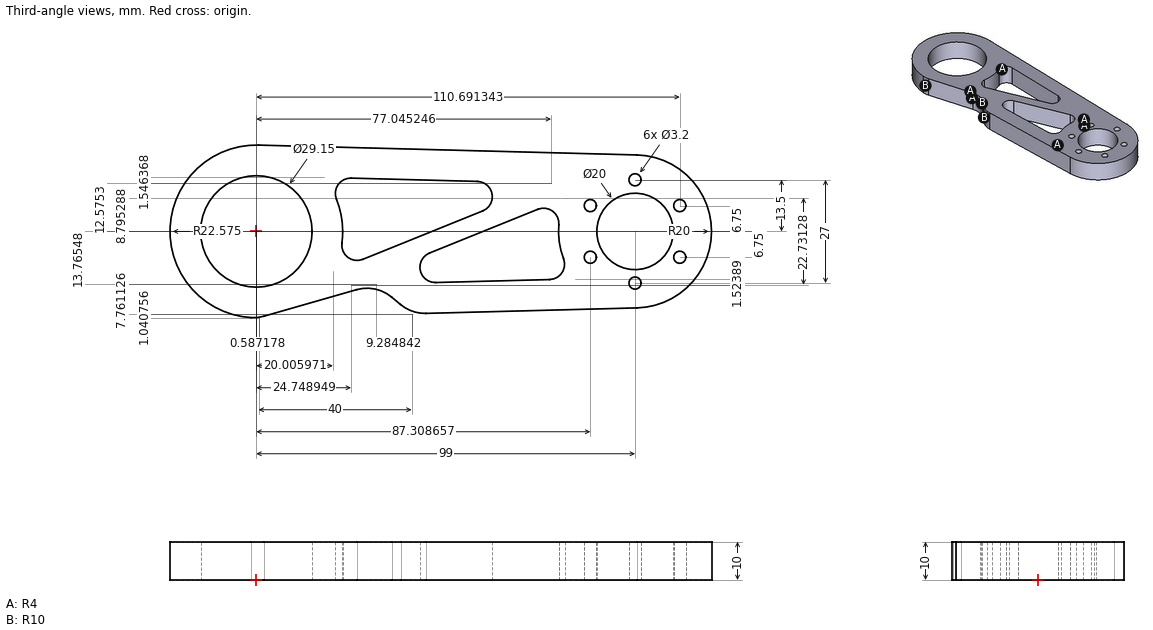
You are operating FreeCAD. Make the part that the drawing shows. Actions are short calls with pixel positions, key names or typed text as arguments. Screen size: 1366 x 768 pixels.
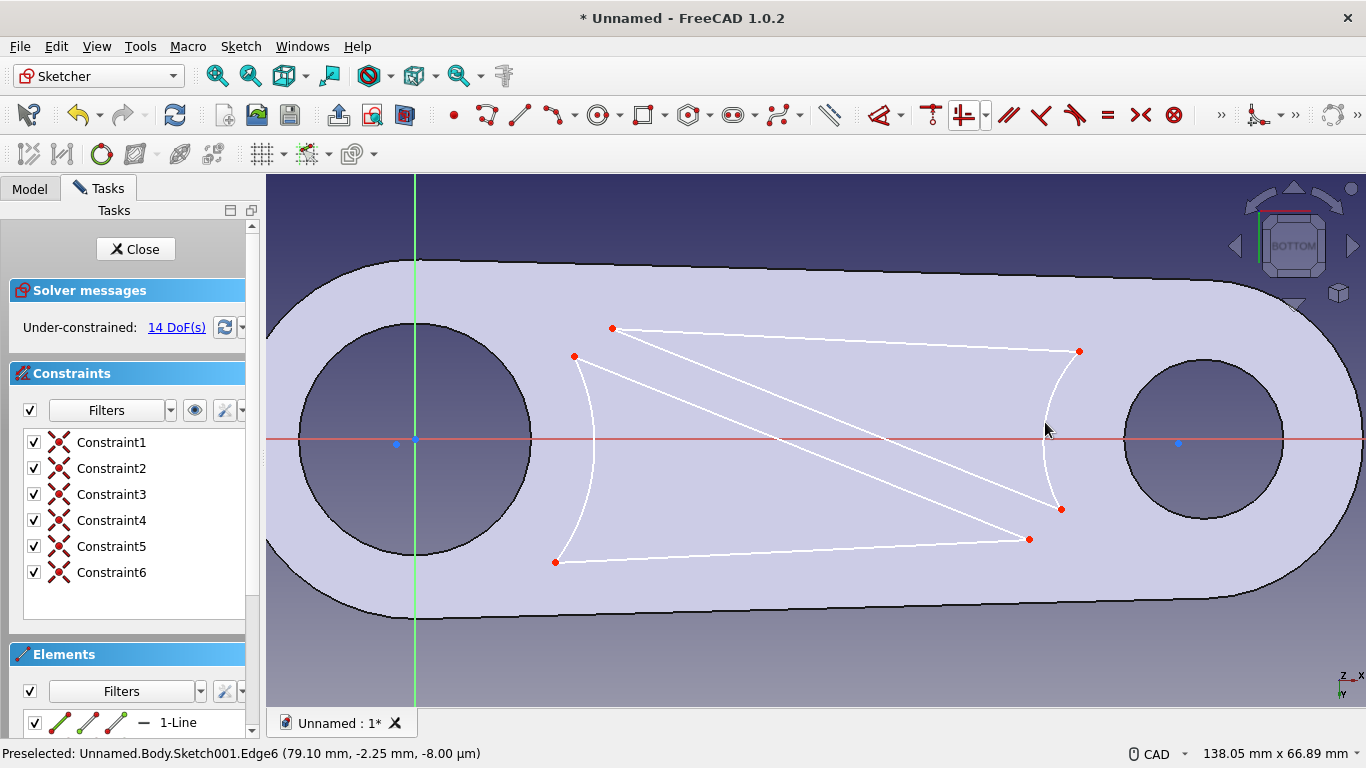
drag(387, 429, 425, 455)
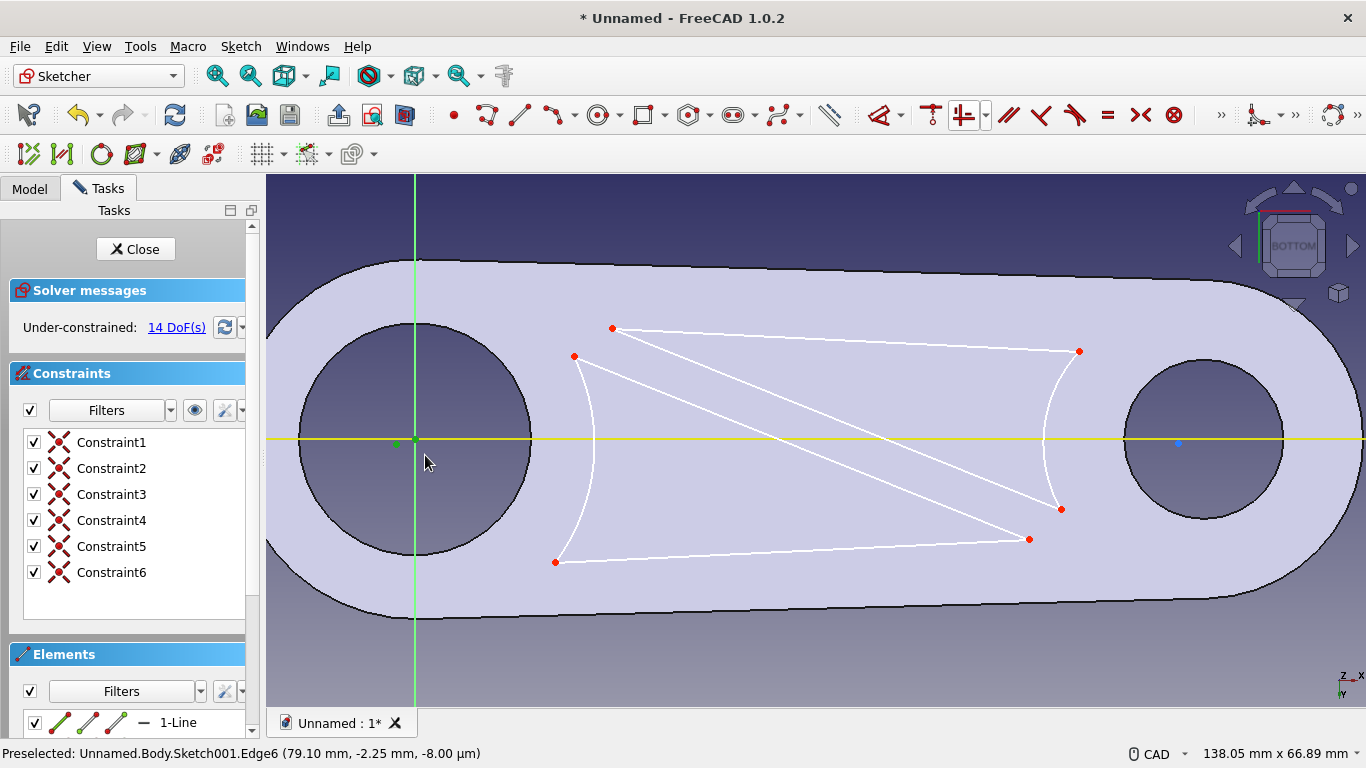
key(c)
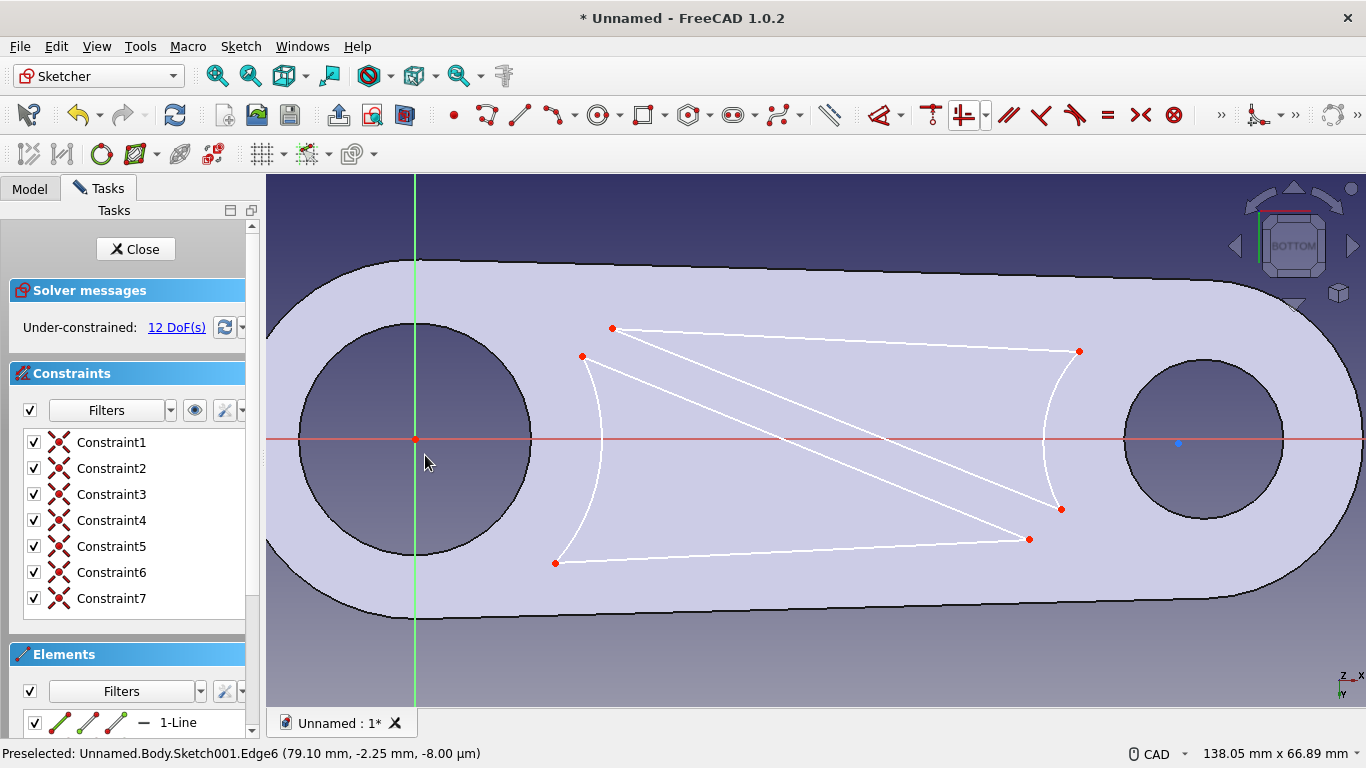
click(1179, 443)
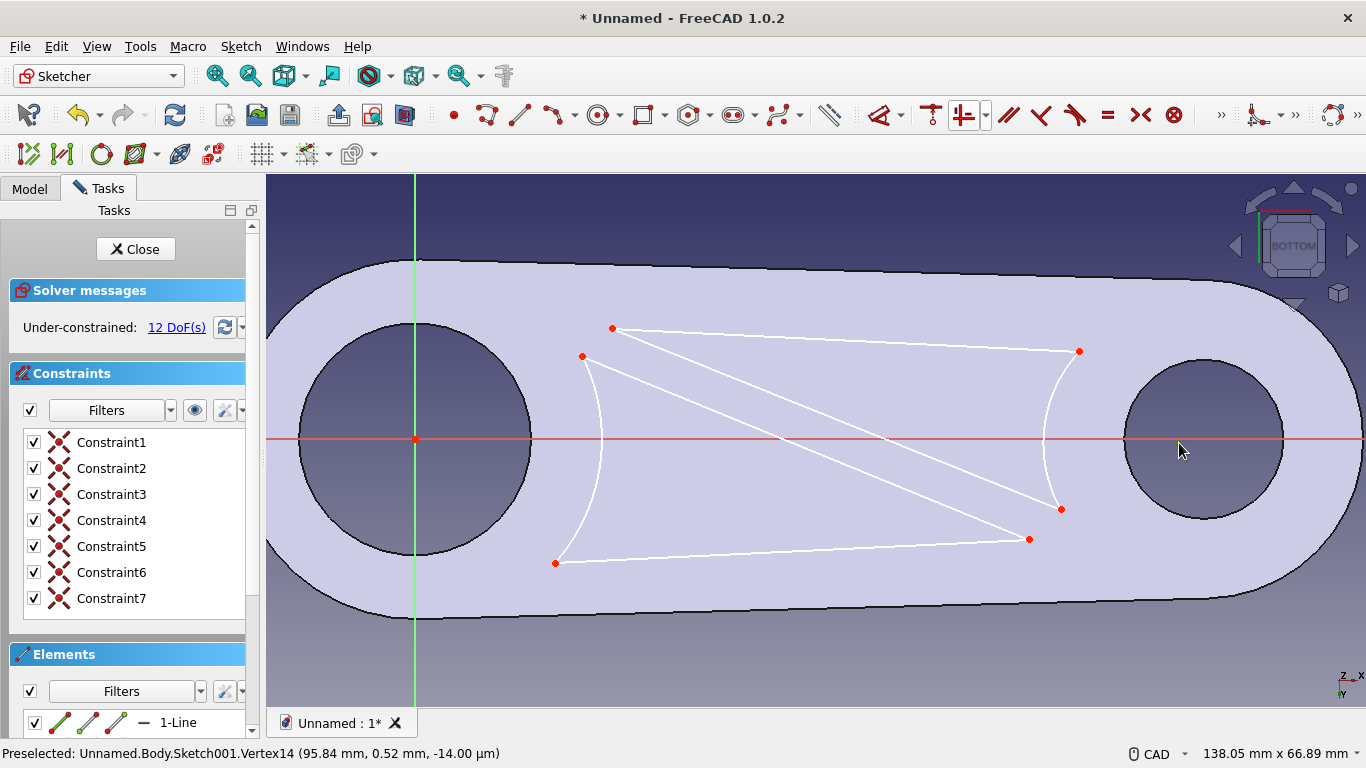
click(359, 439)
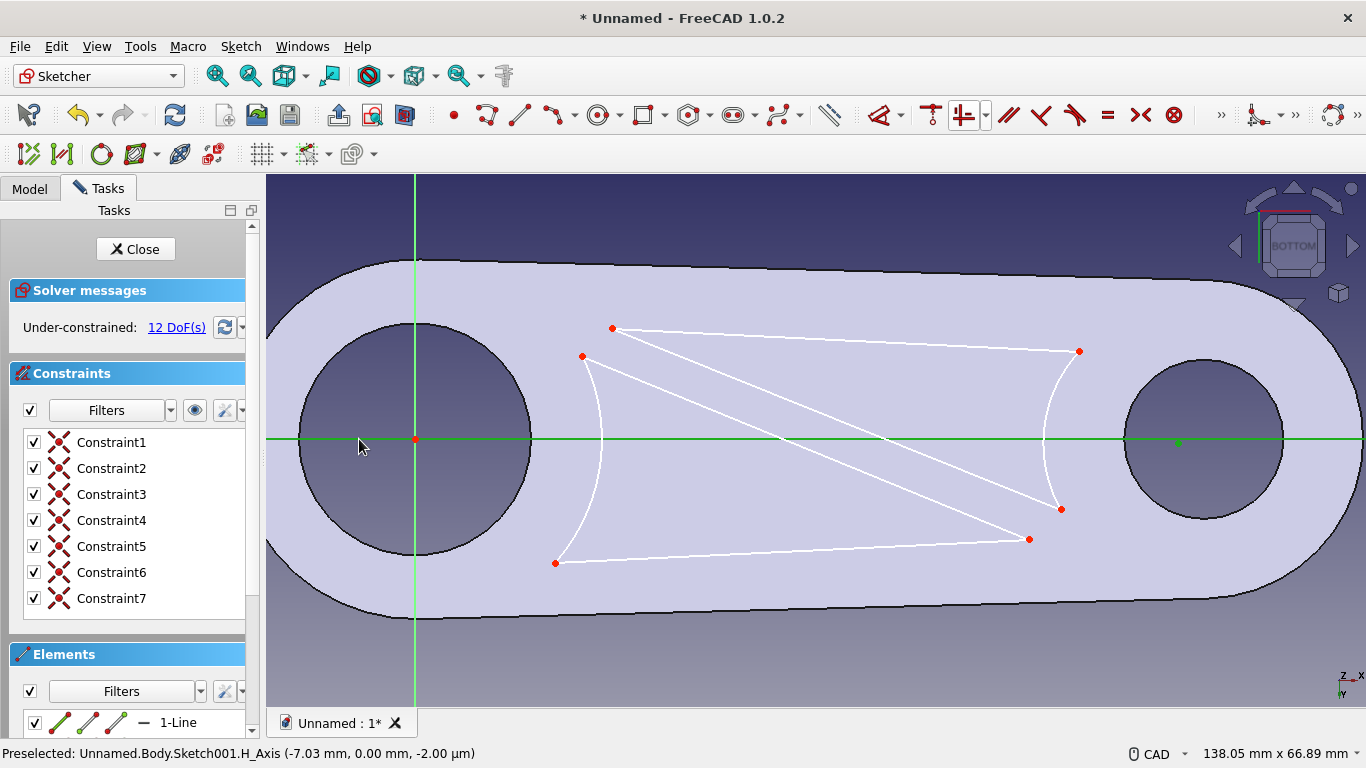
key(c)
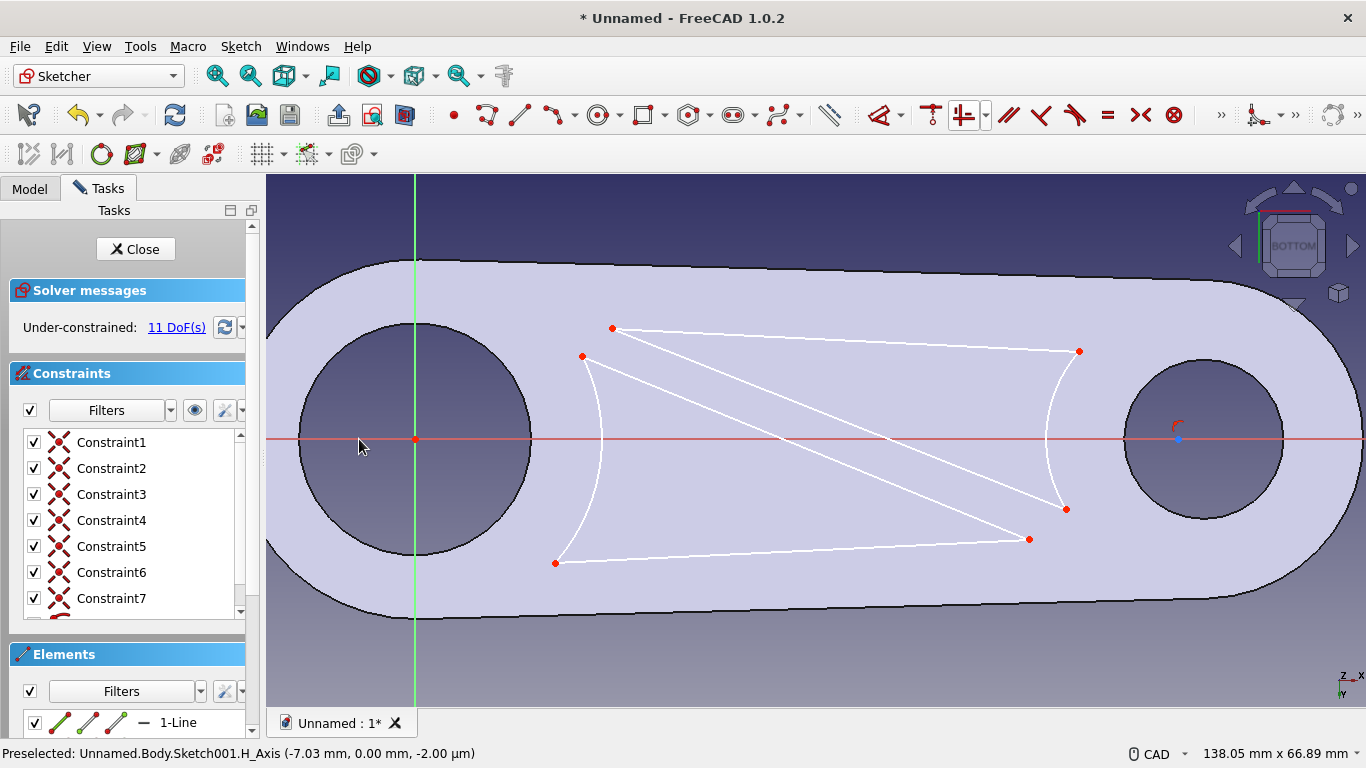
click(878, 116)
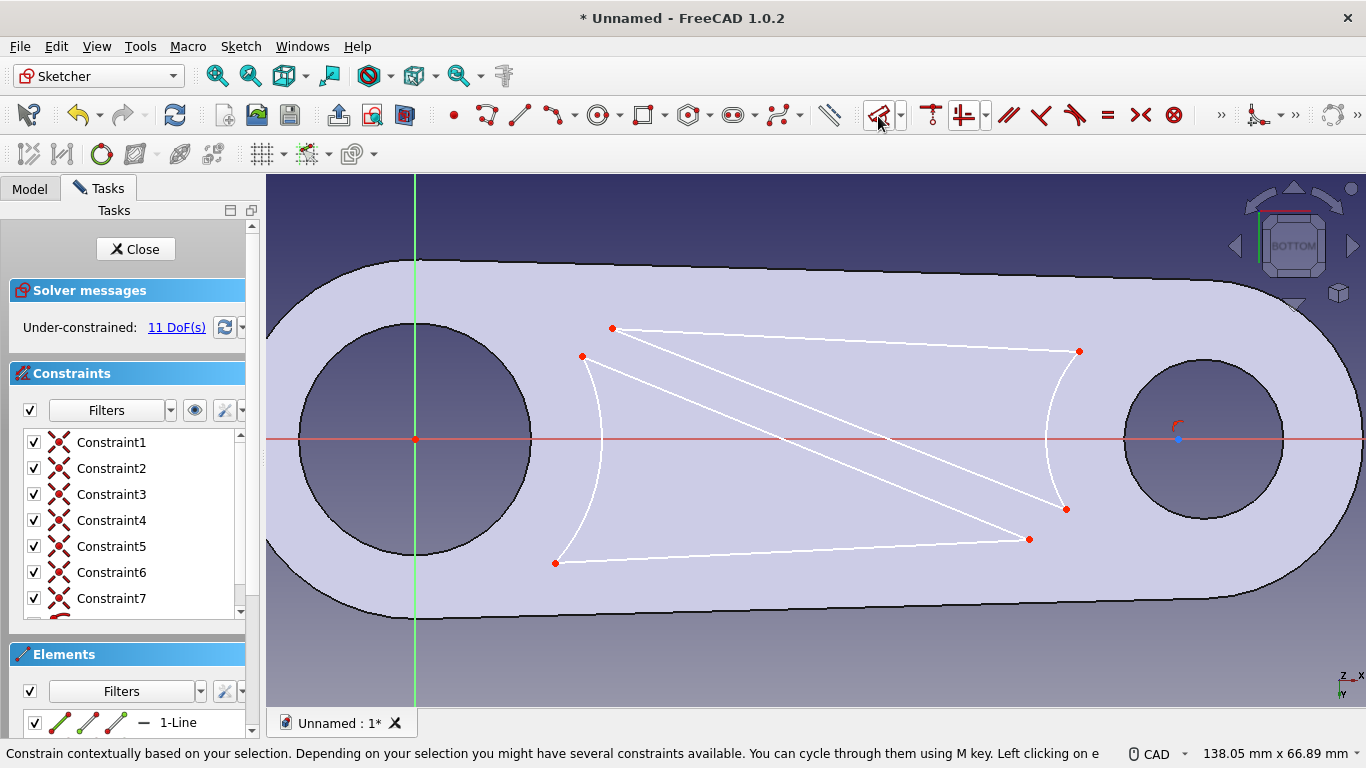
click(589, 507)
click(619, 519)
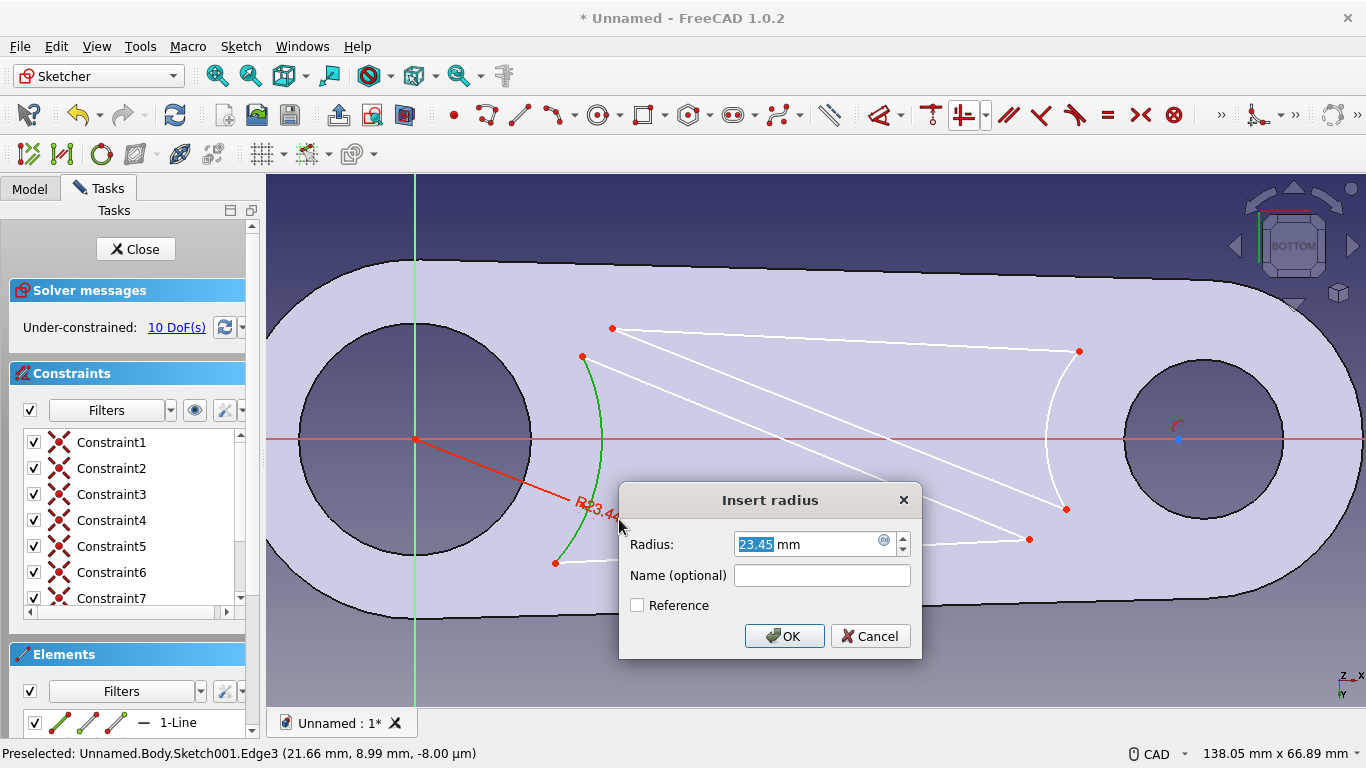
text(22.575)
key(Return)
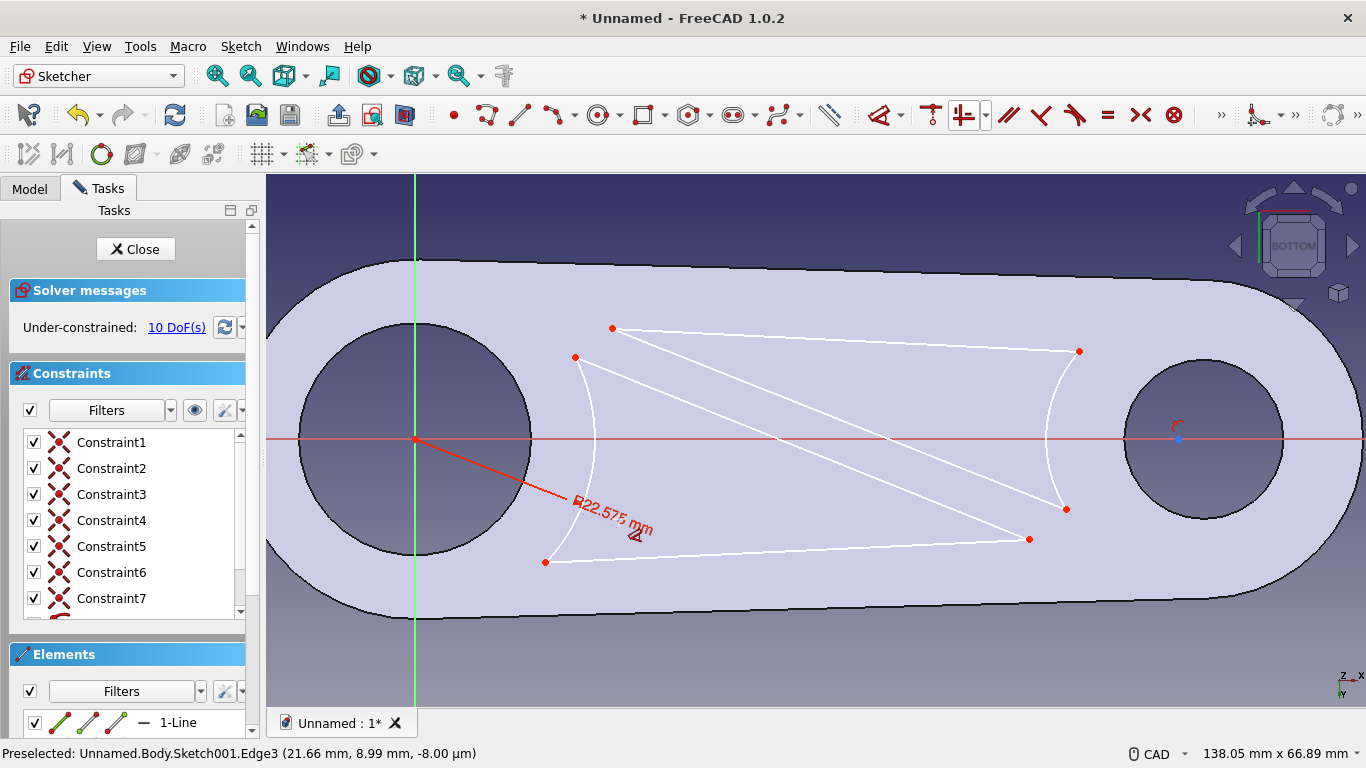
click(1054, 396)
click(1024, 386)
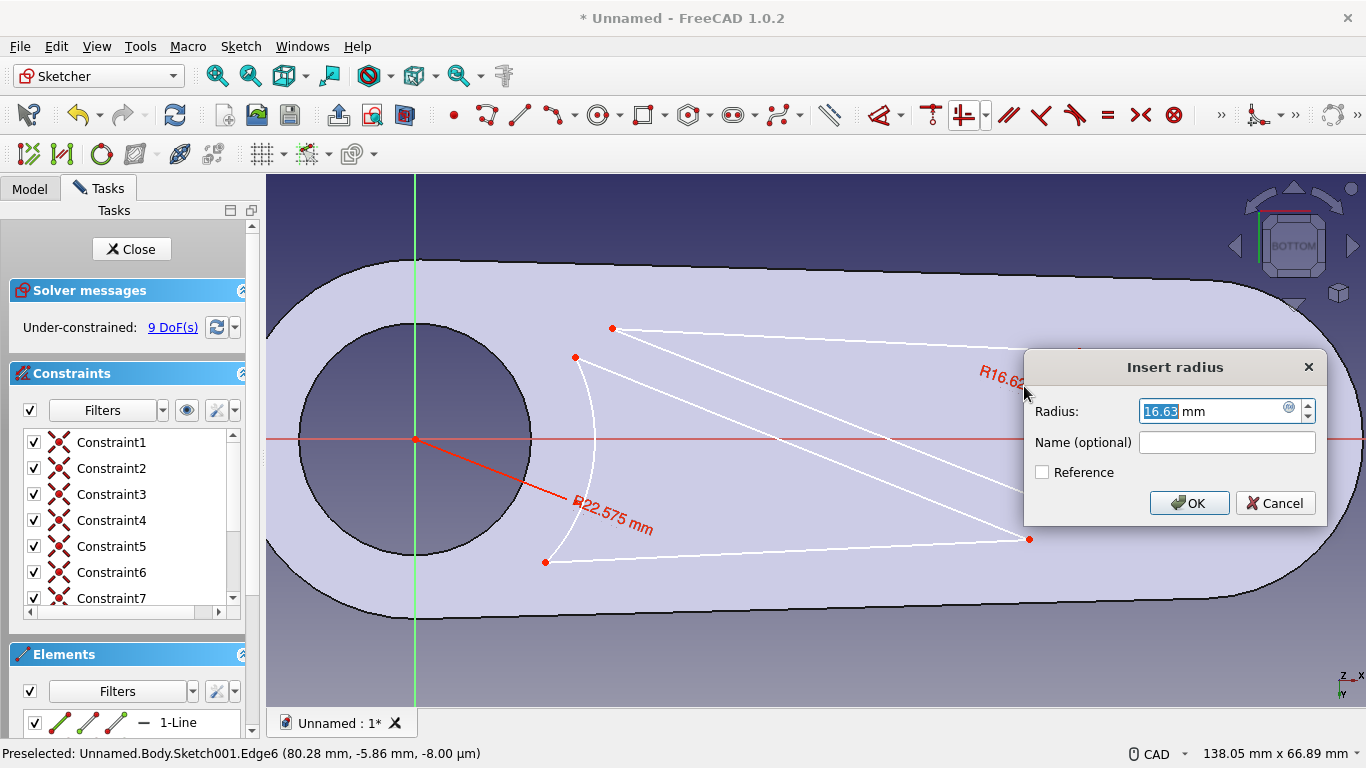
text(20)
key(Return)